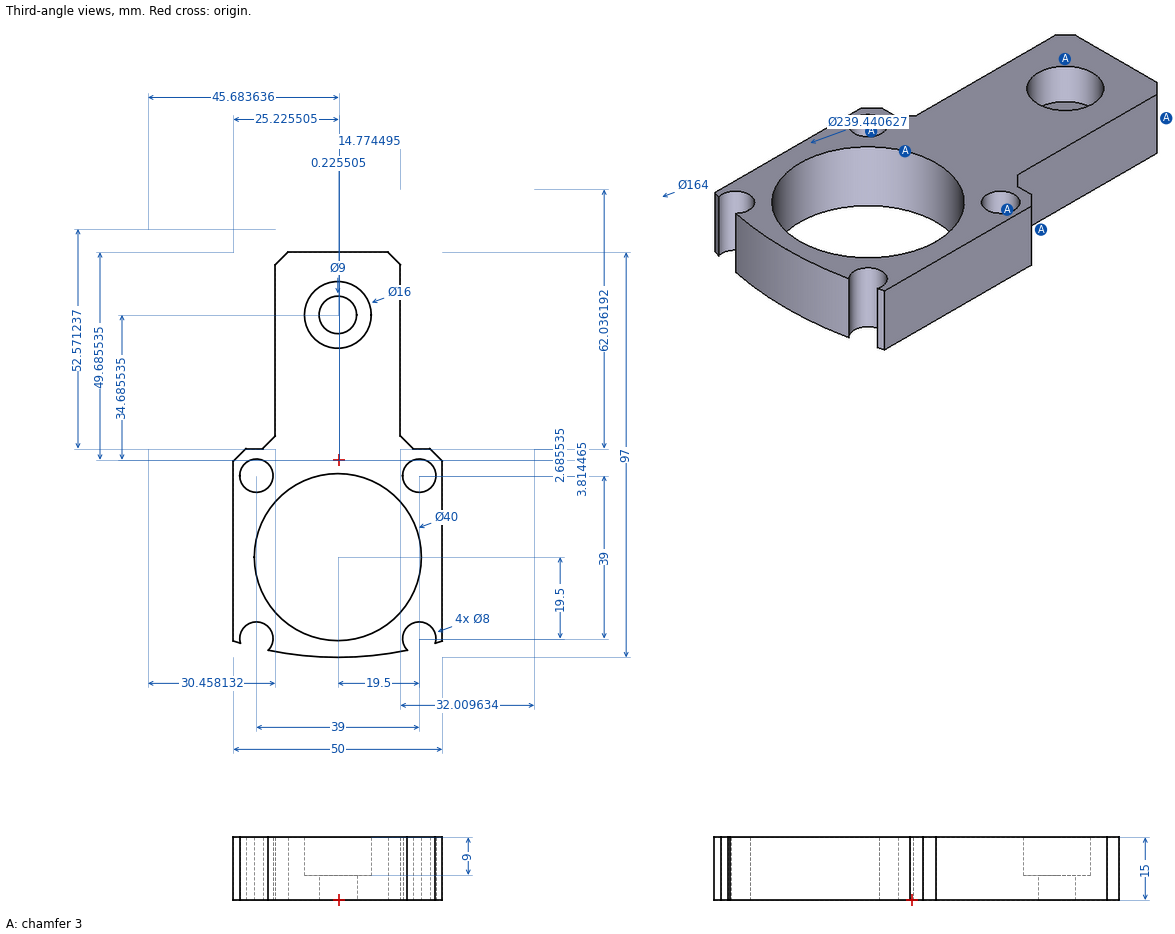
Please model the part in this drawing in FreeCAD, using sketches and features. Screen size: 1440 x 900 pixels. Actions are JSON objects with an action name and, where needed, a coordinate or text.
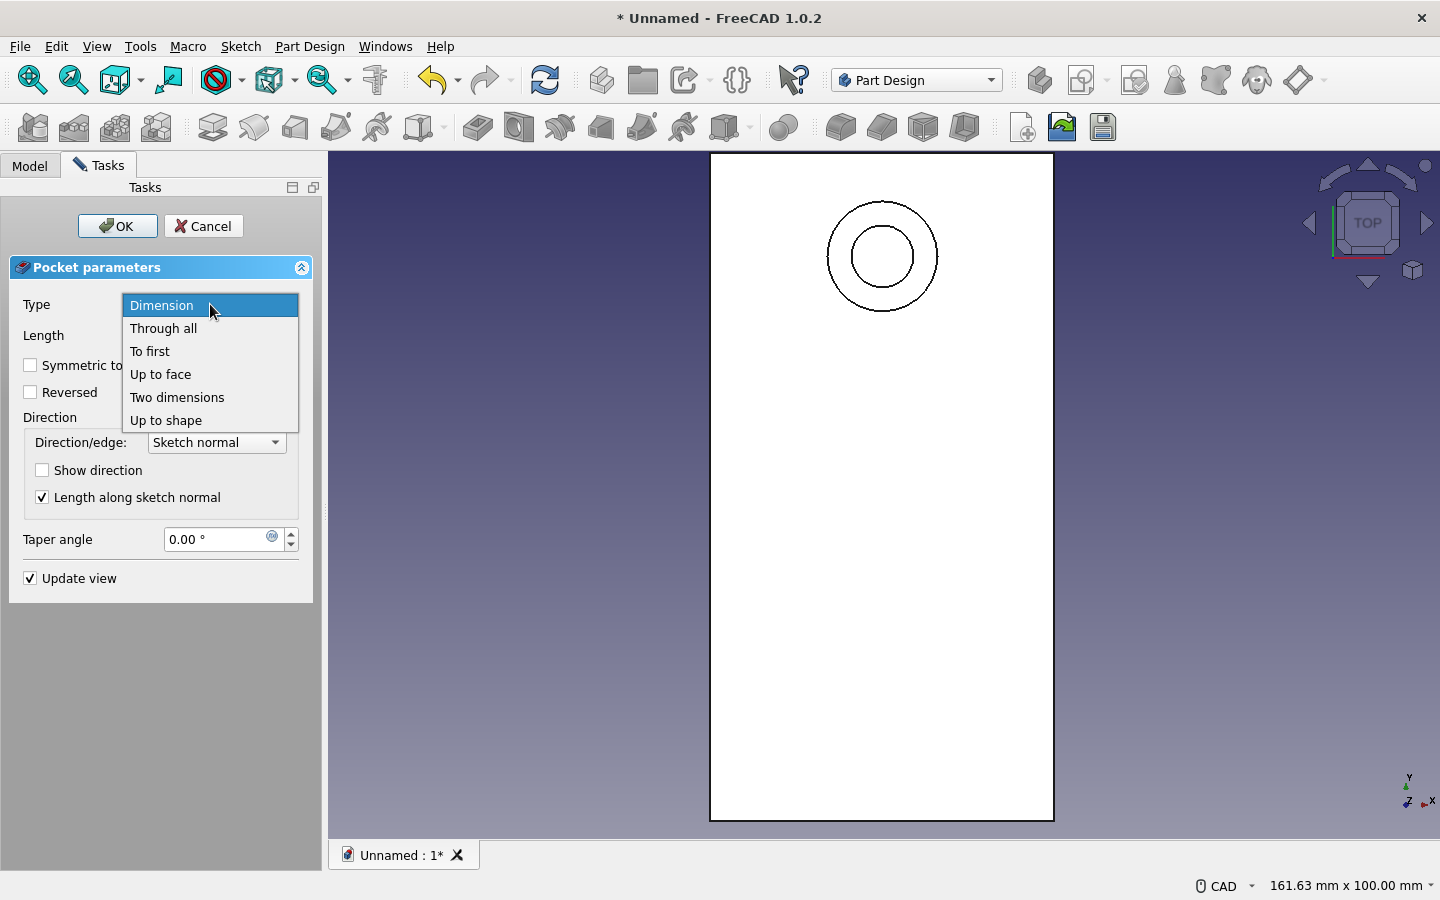
{"action": "left_click", "coordinate": [208, 328]}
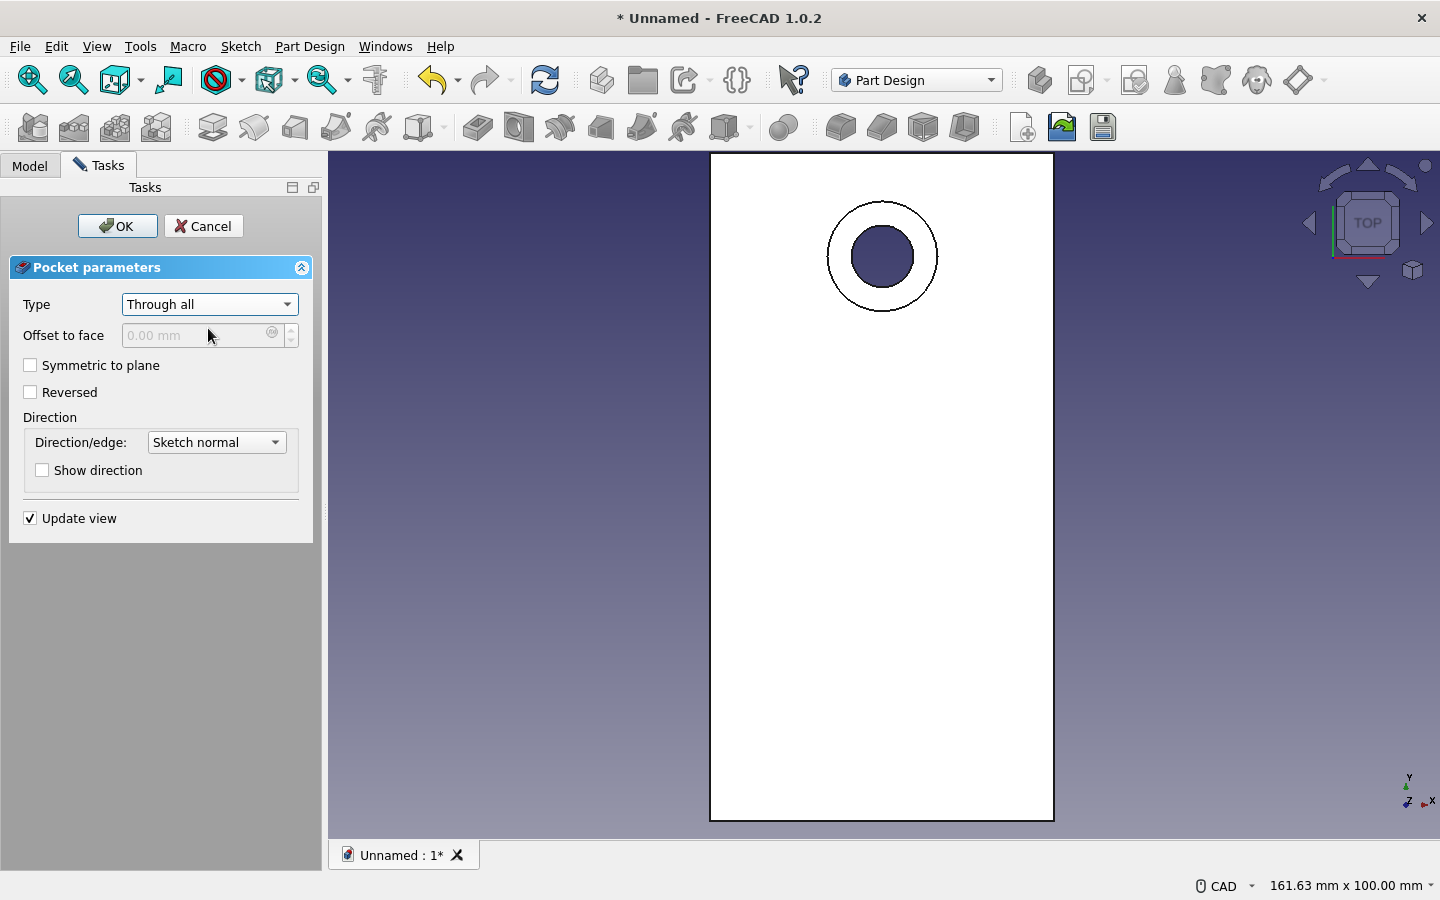
{"action": "left_click", "coordinate": [118, 226]}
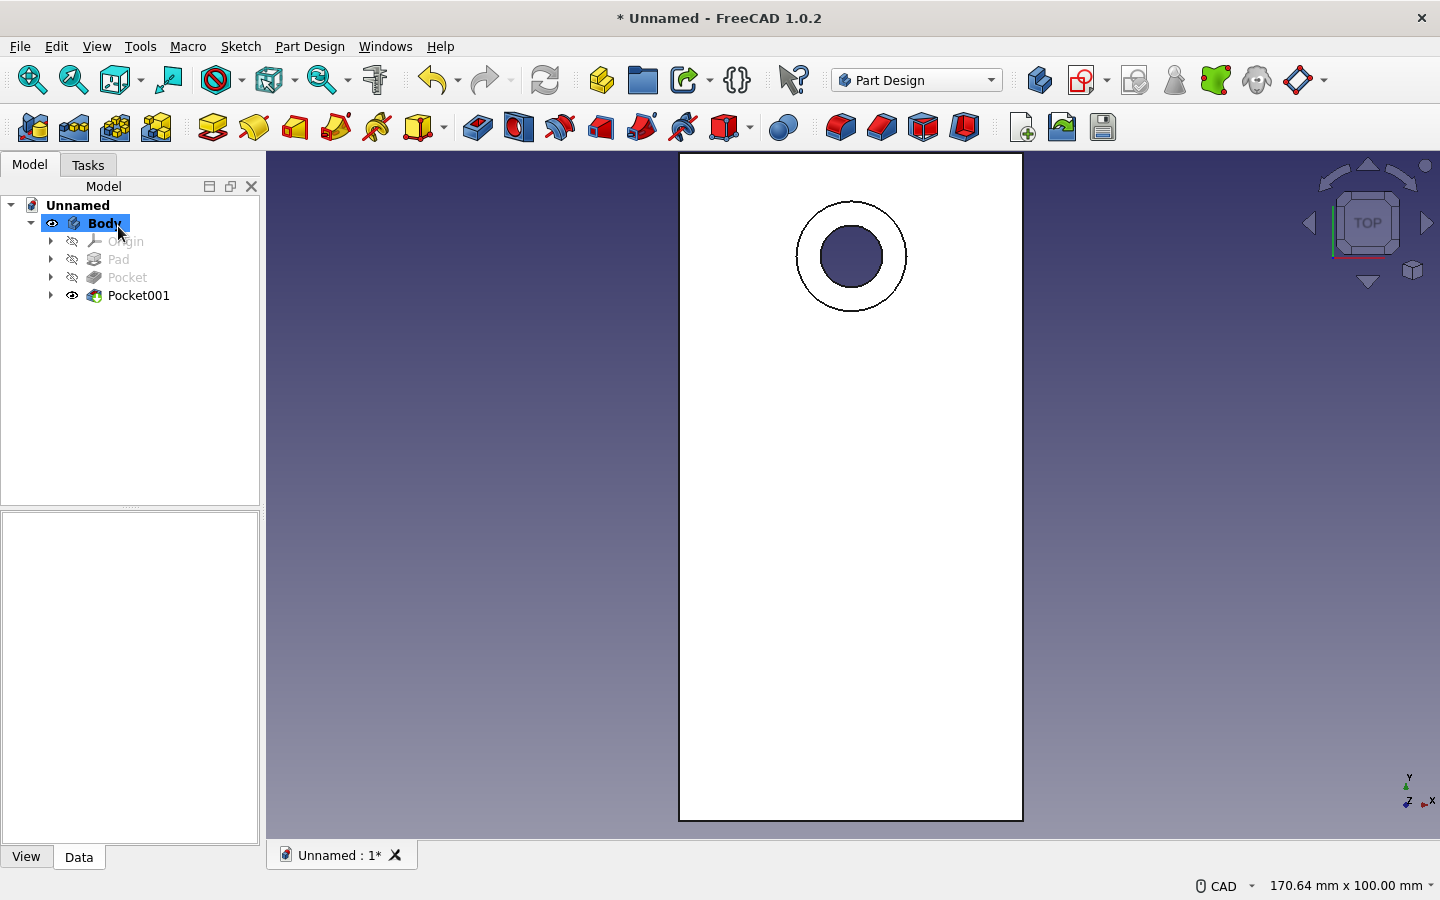
{"action": "key", "text": "5"}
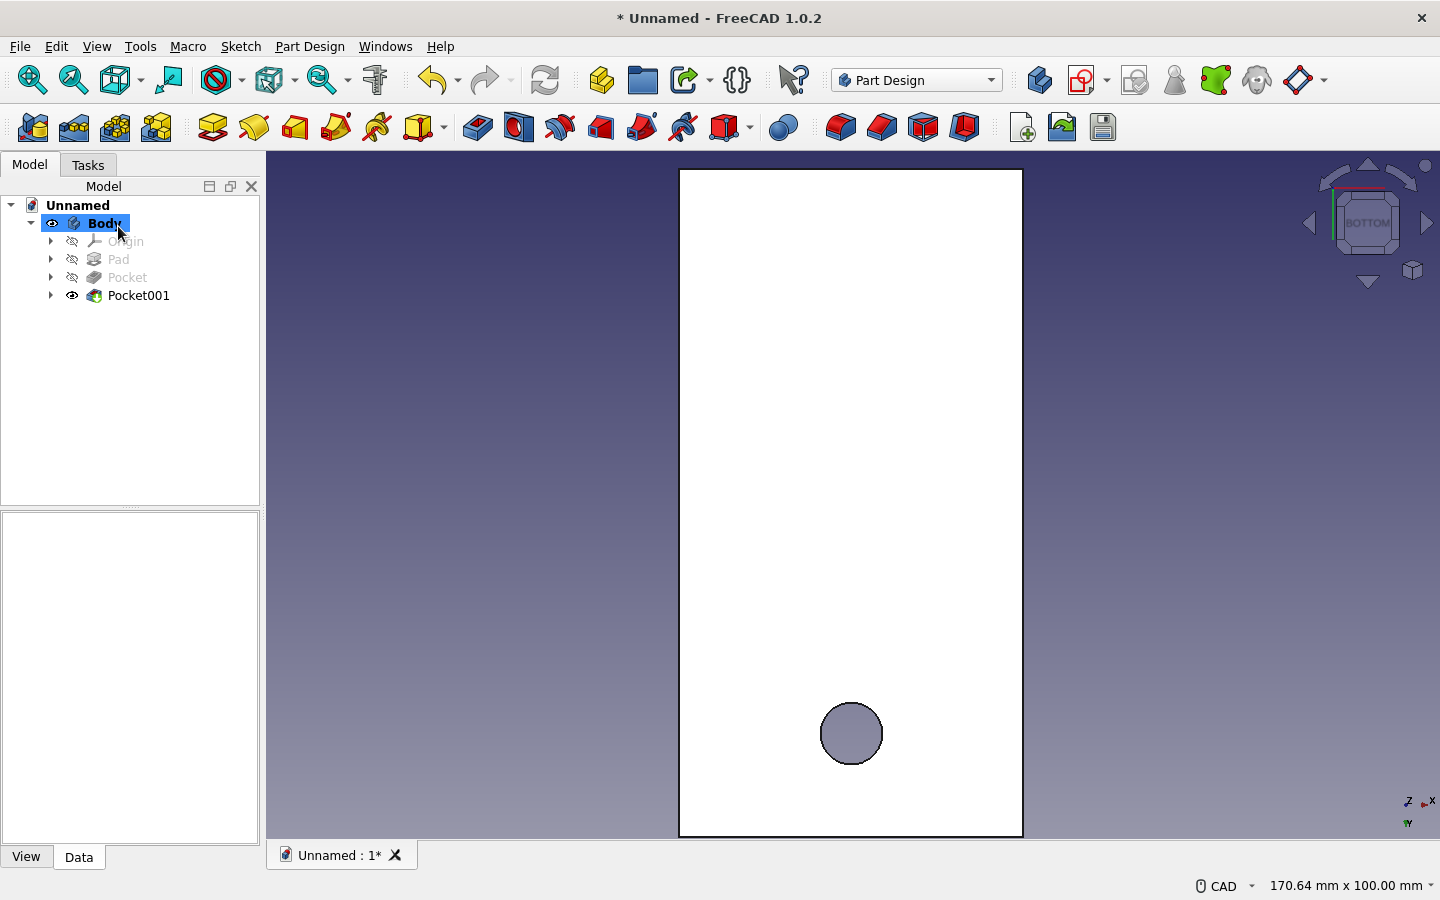
{"action": "left_click", "coordinate": [851, 502]}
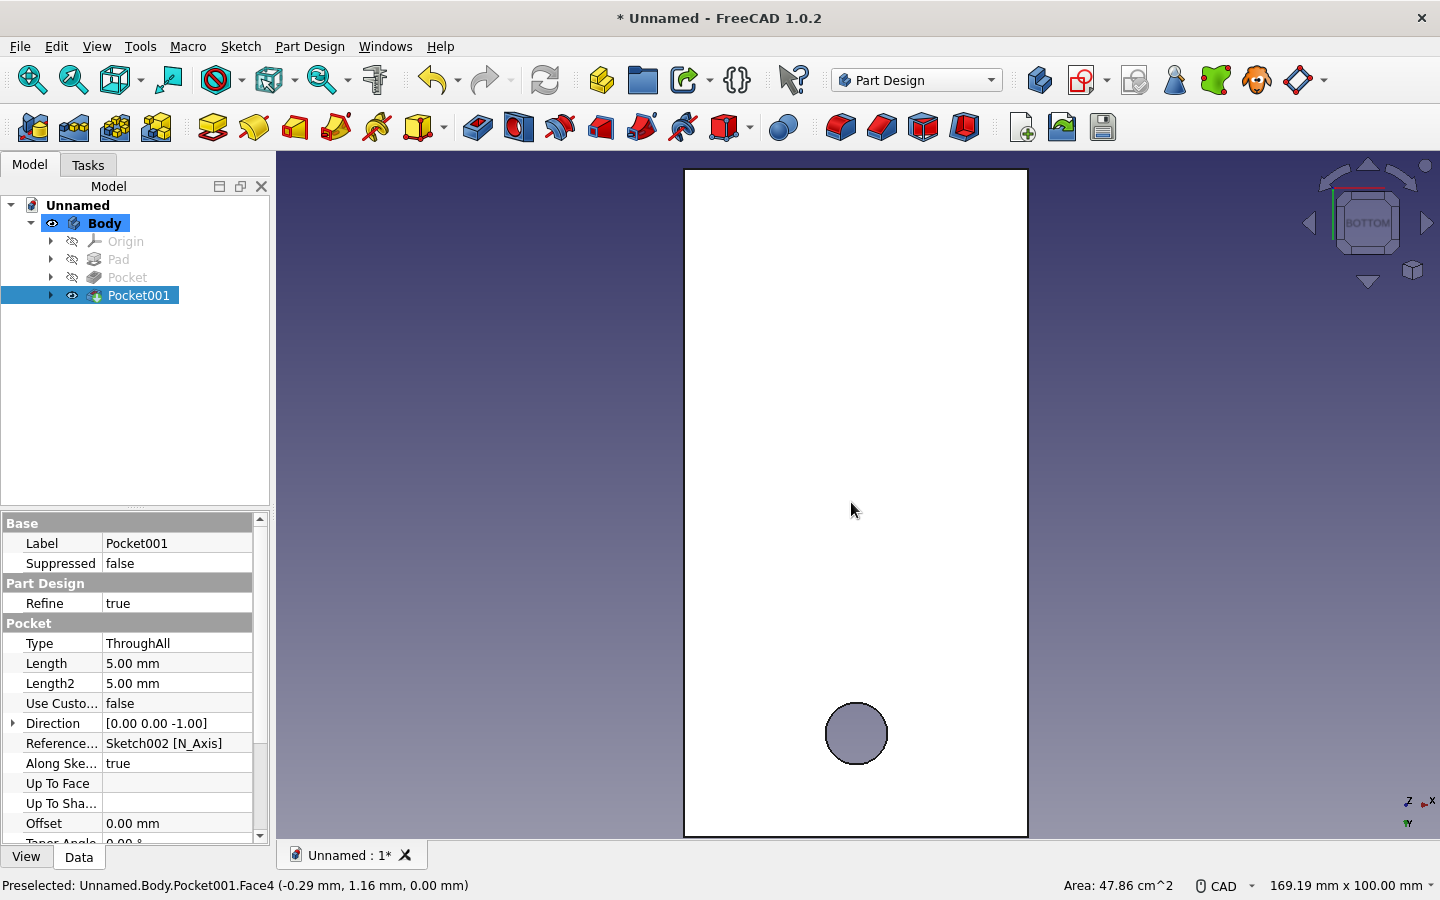
{"action": "left_click", "coordinate": [1080, 80]}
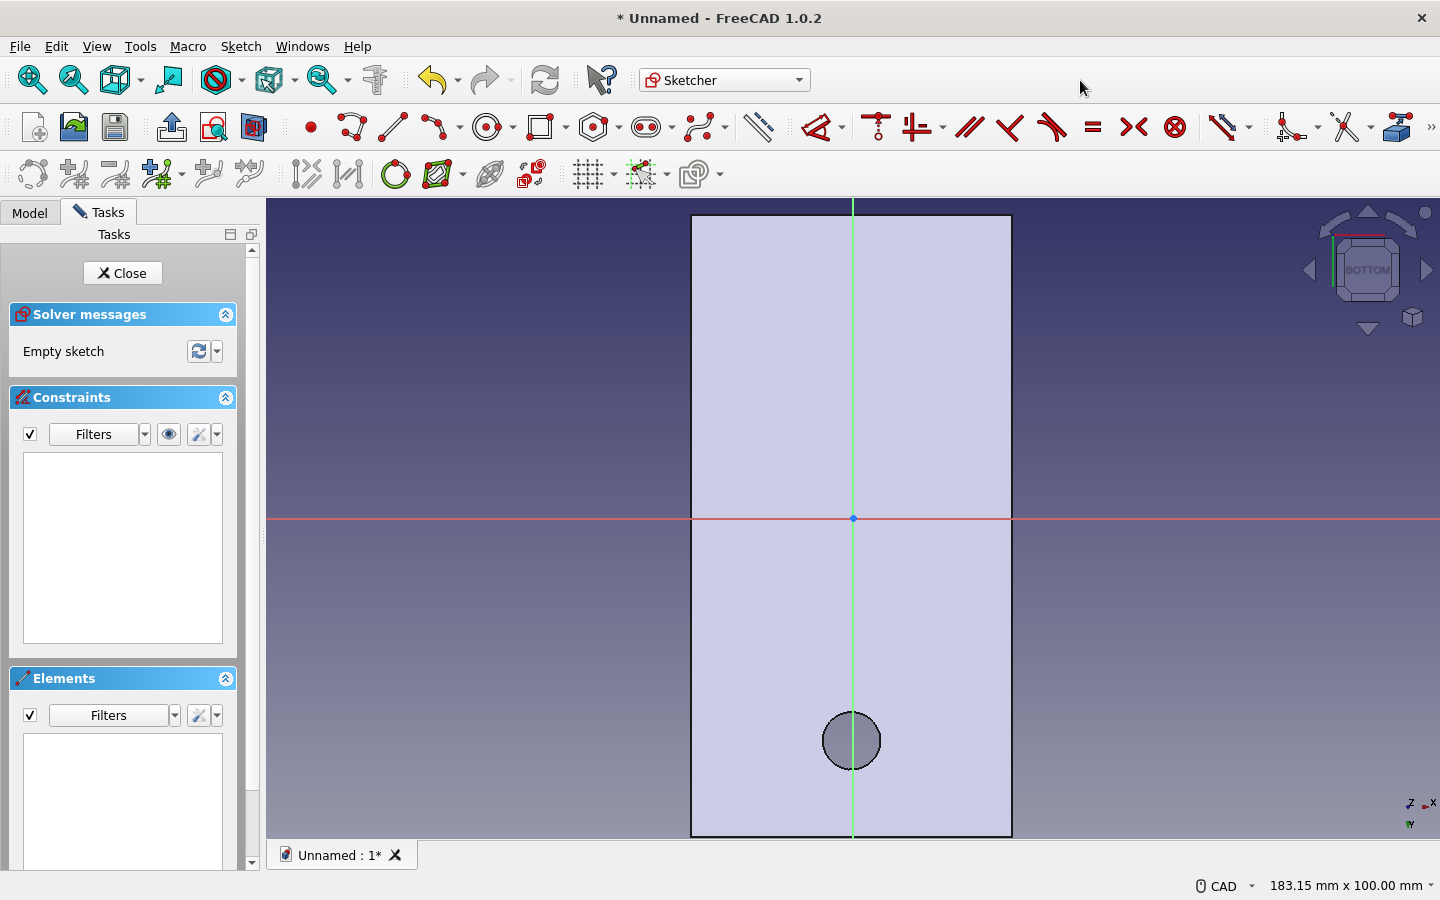
{"action": "scroll", "coordinate": [482, 811], "scroll_direction": "down", "scroll_amount": 1}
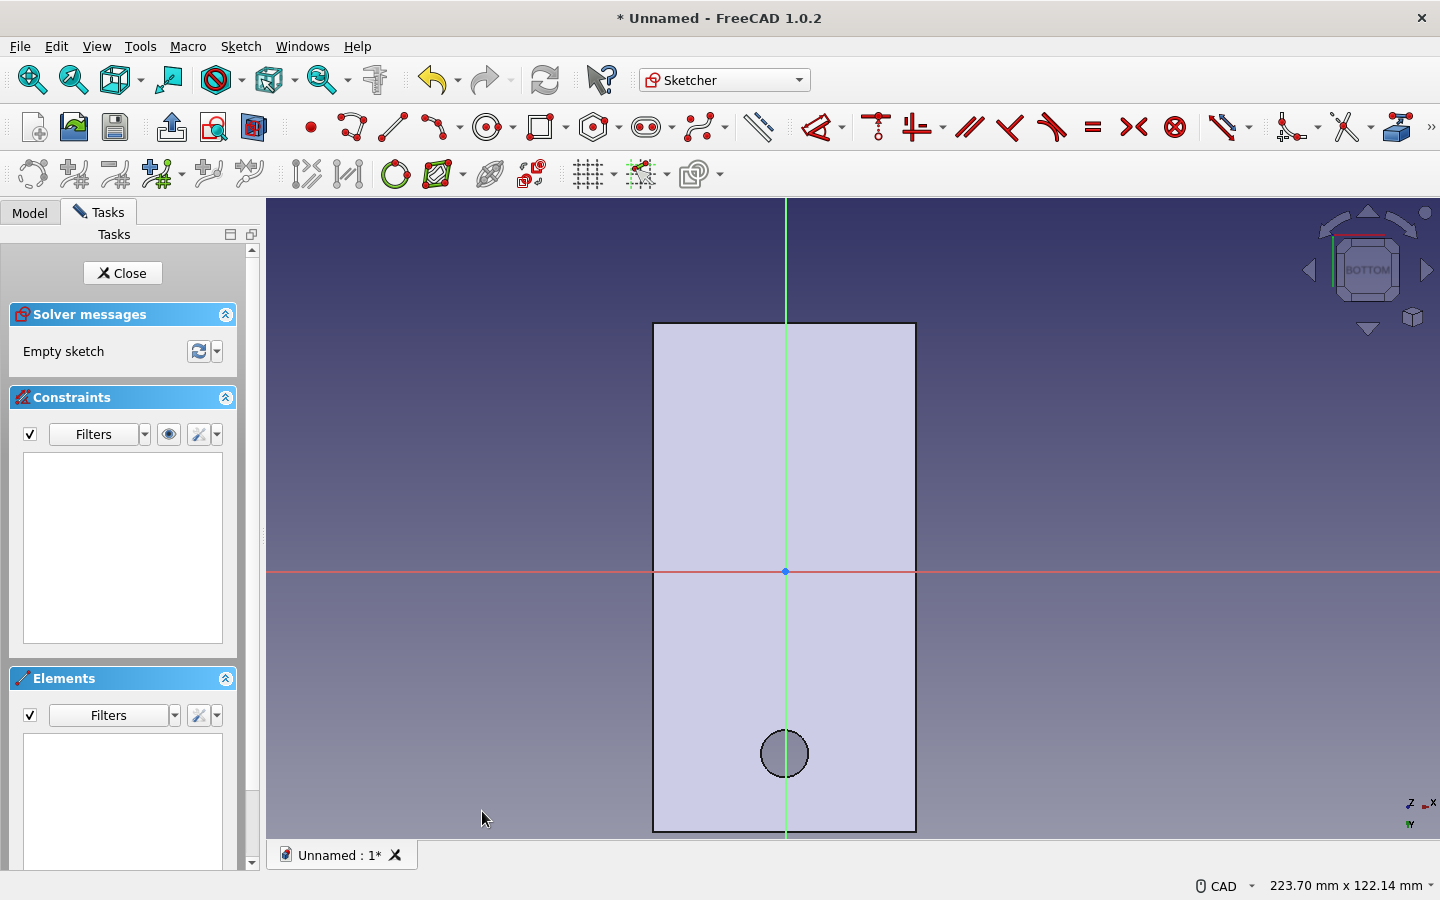
{"action": "scroll", "coordinate": [785, 365], "scroll_direction": "up", "scroll_amount": 3}